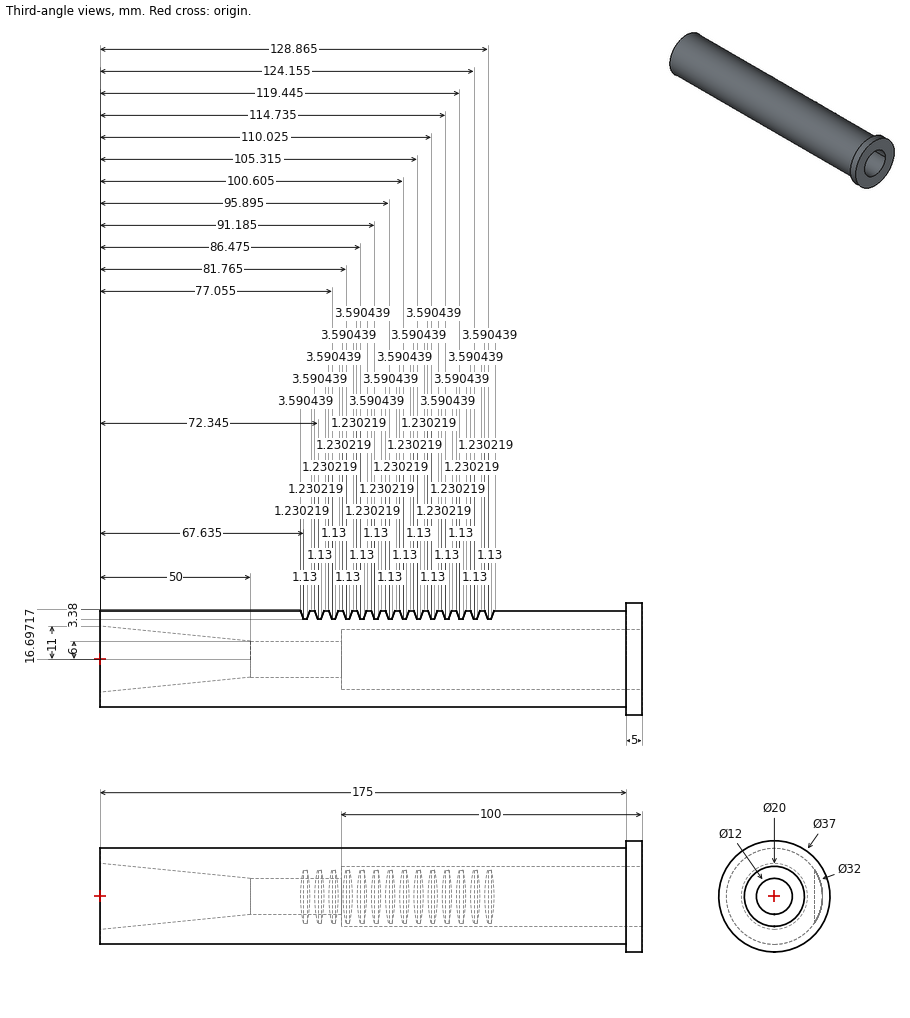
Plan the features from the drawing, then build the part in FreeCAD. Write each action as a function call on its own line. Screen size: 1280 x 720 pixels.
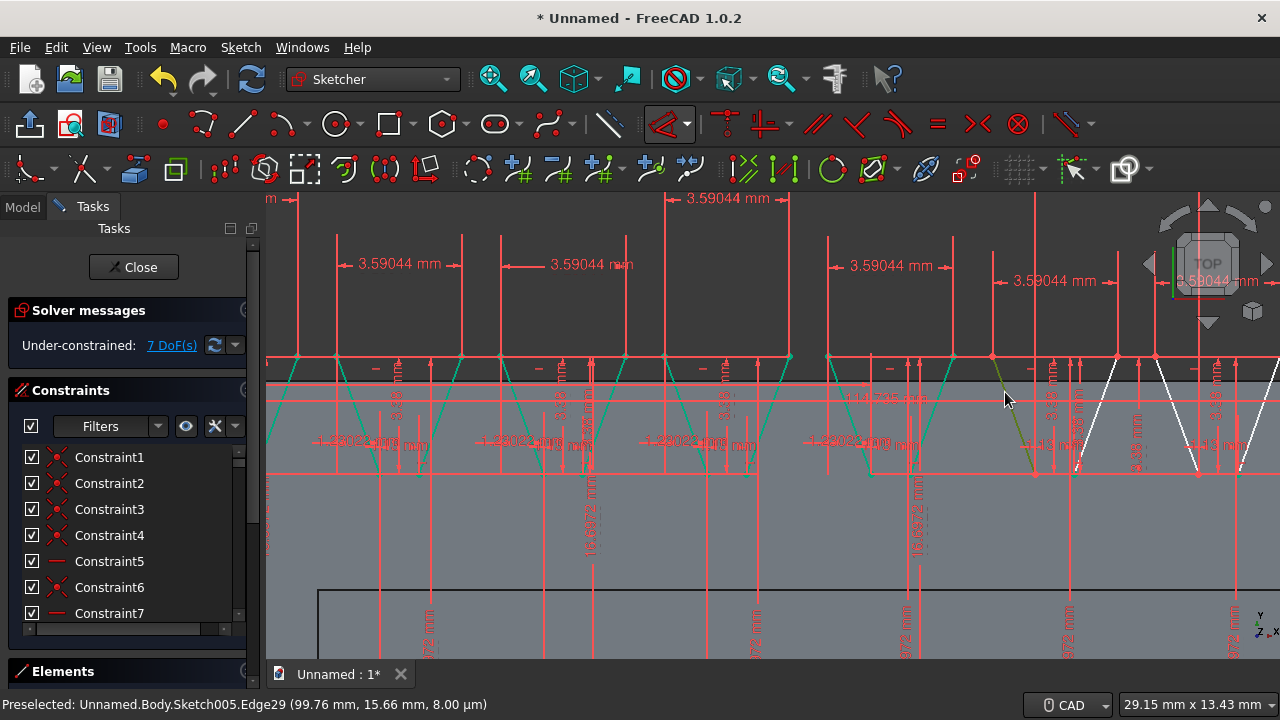
click(690, 124)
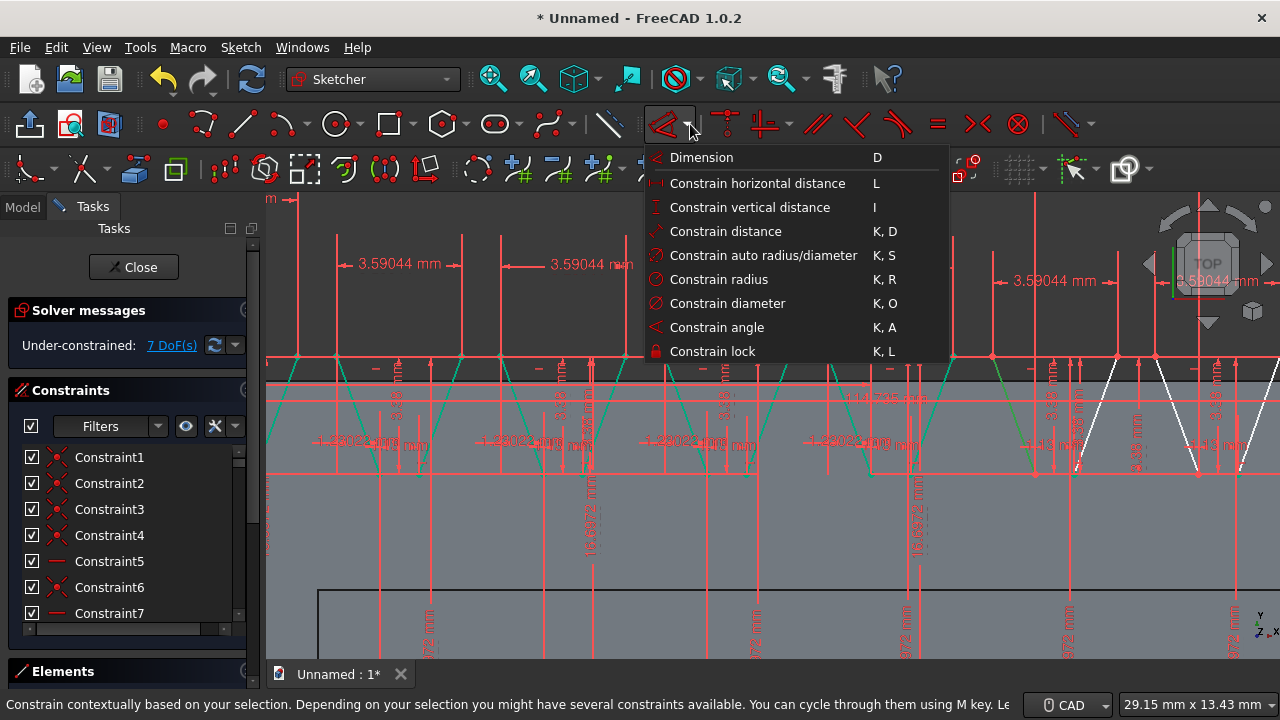
click(797, 183)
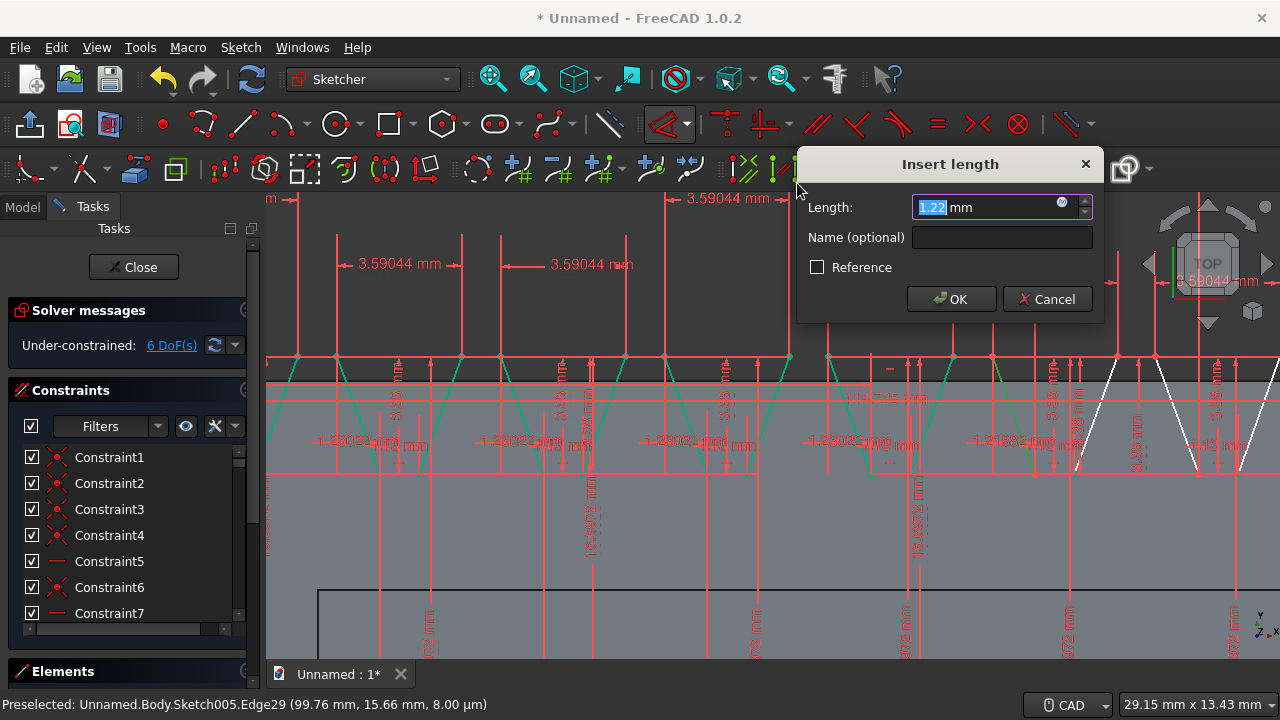
text(1.230219)
key(Return)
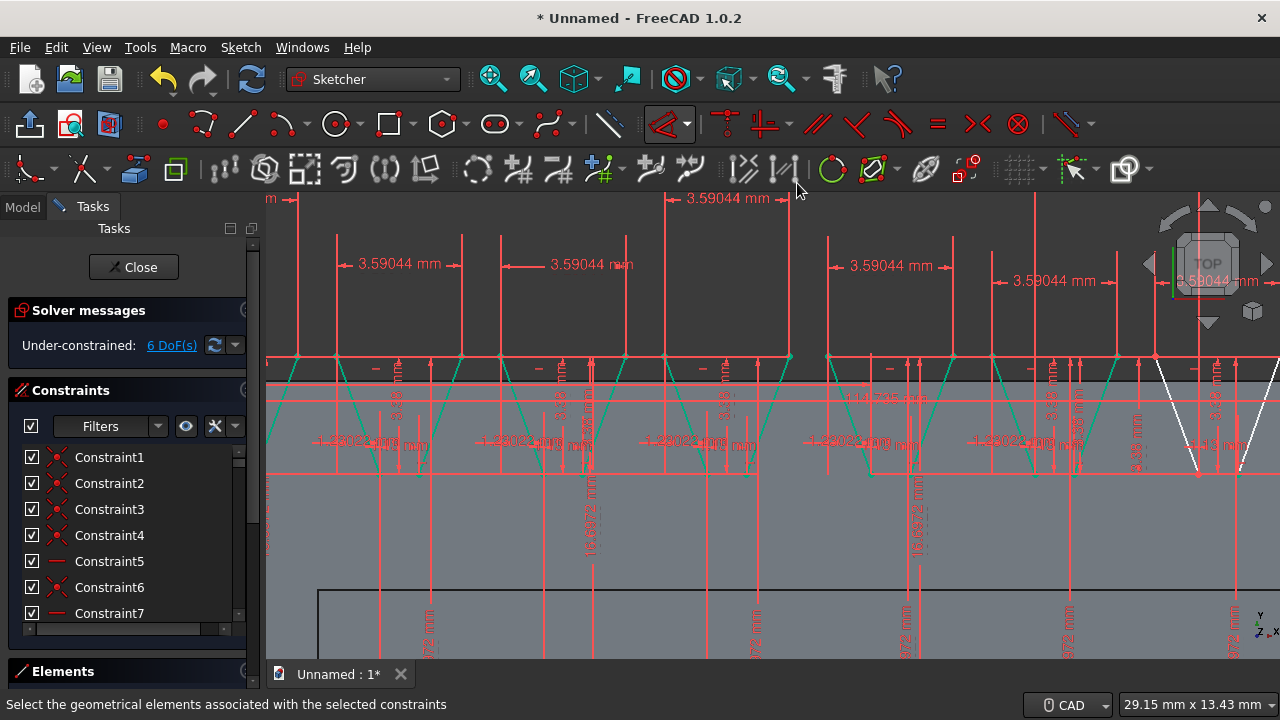
scroll(843, 391, down, 10)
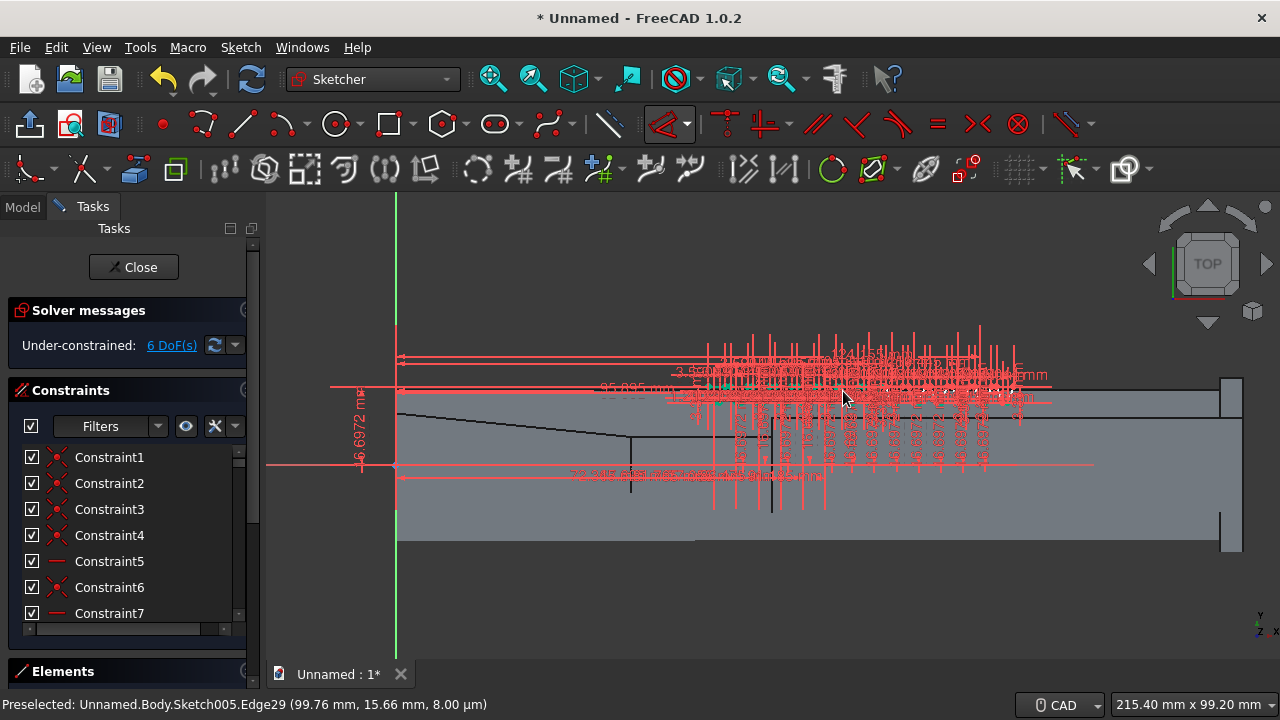
scroll(888, 391, up, 10)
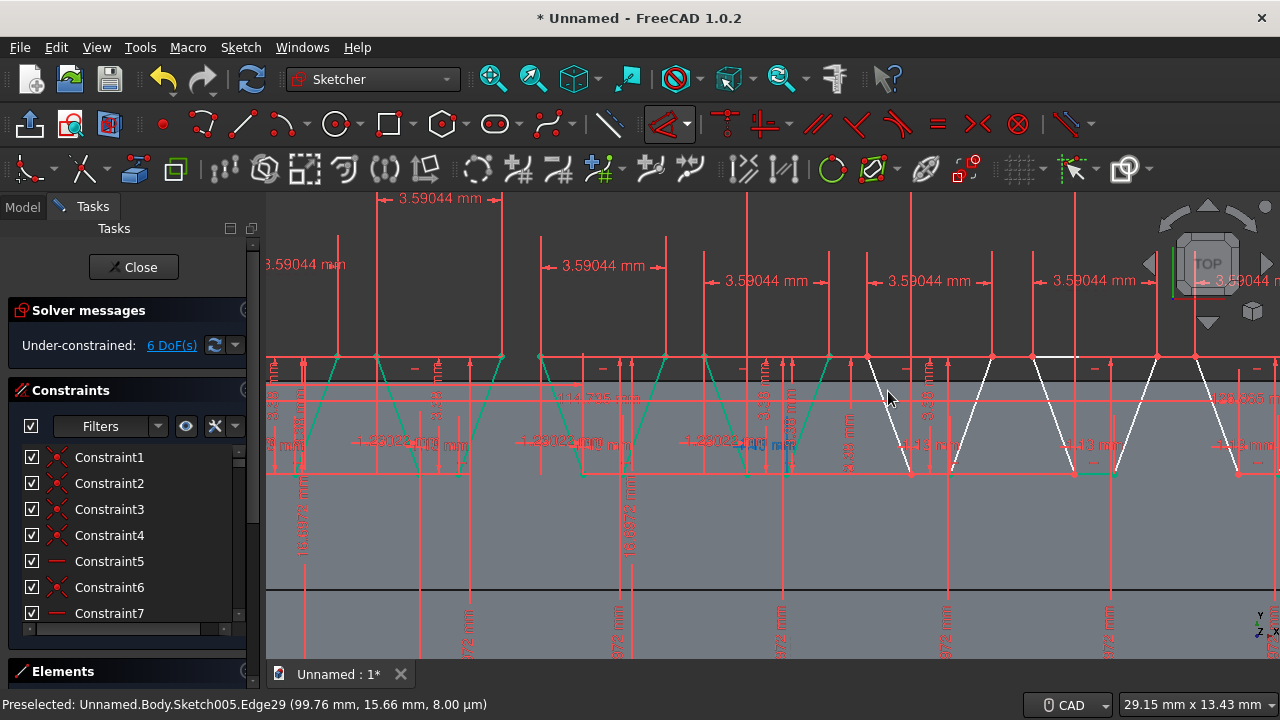
click(880, 392)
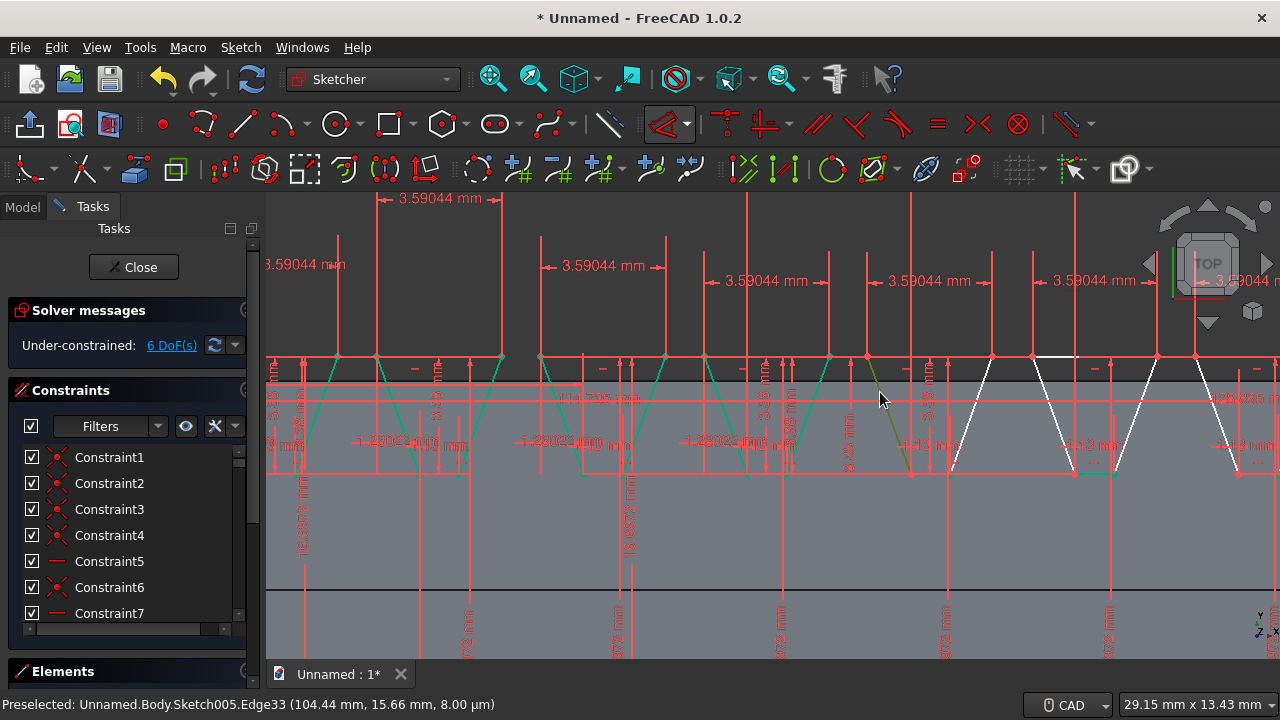
key(l)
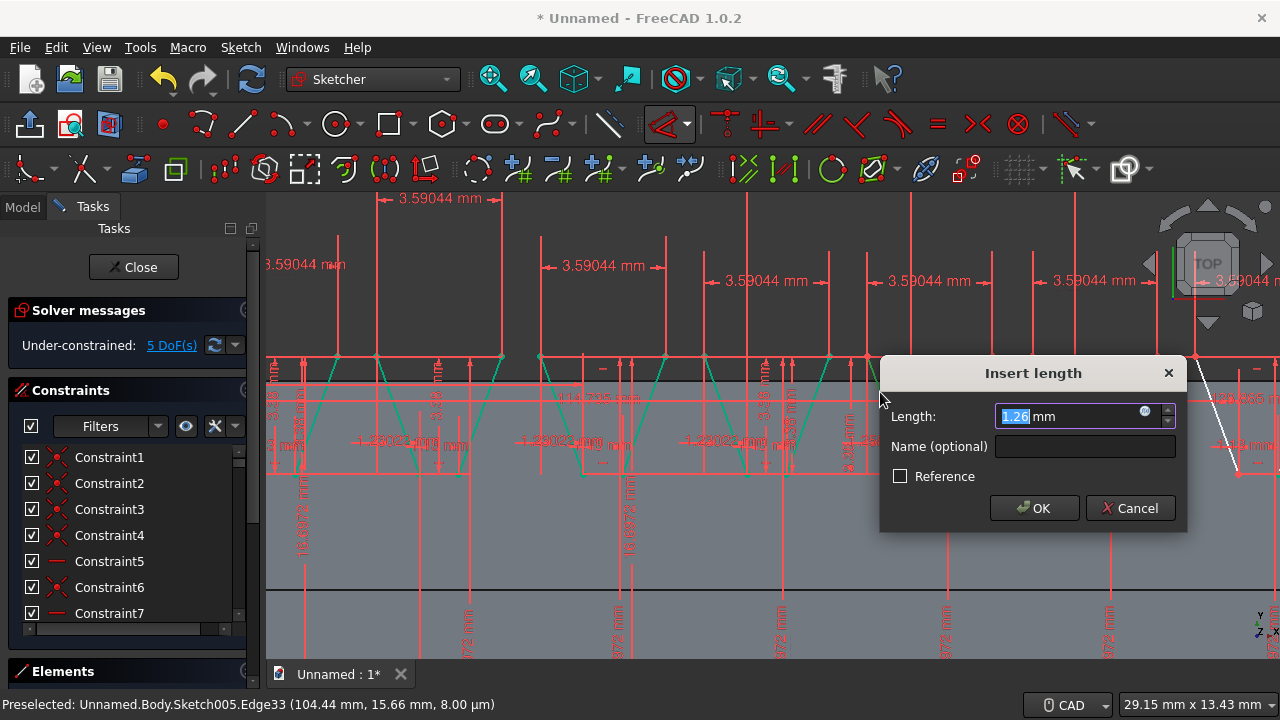
text(1.230219)
key(Return)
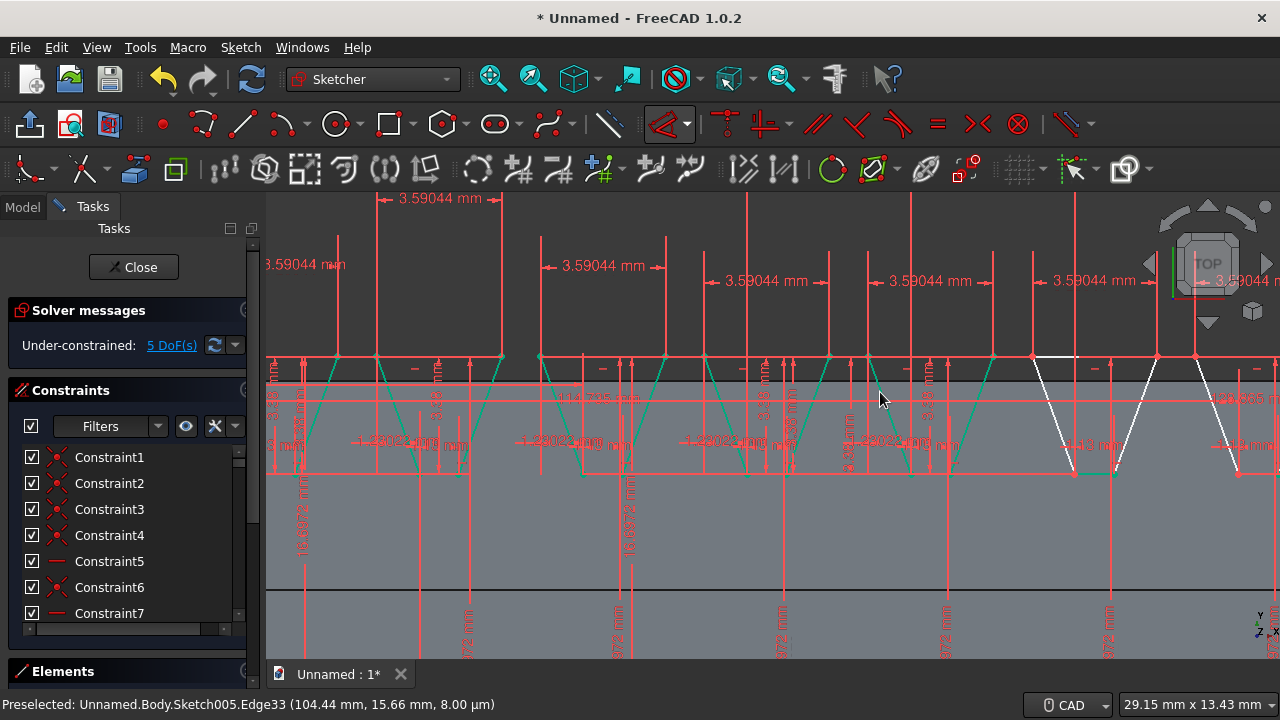
click(1045, 392)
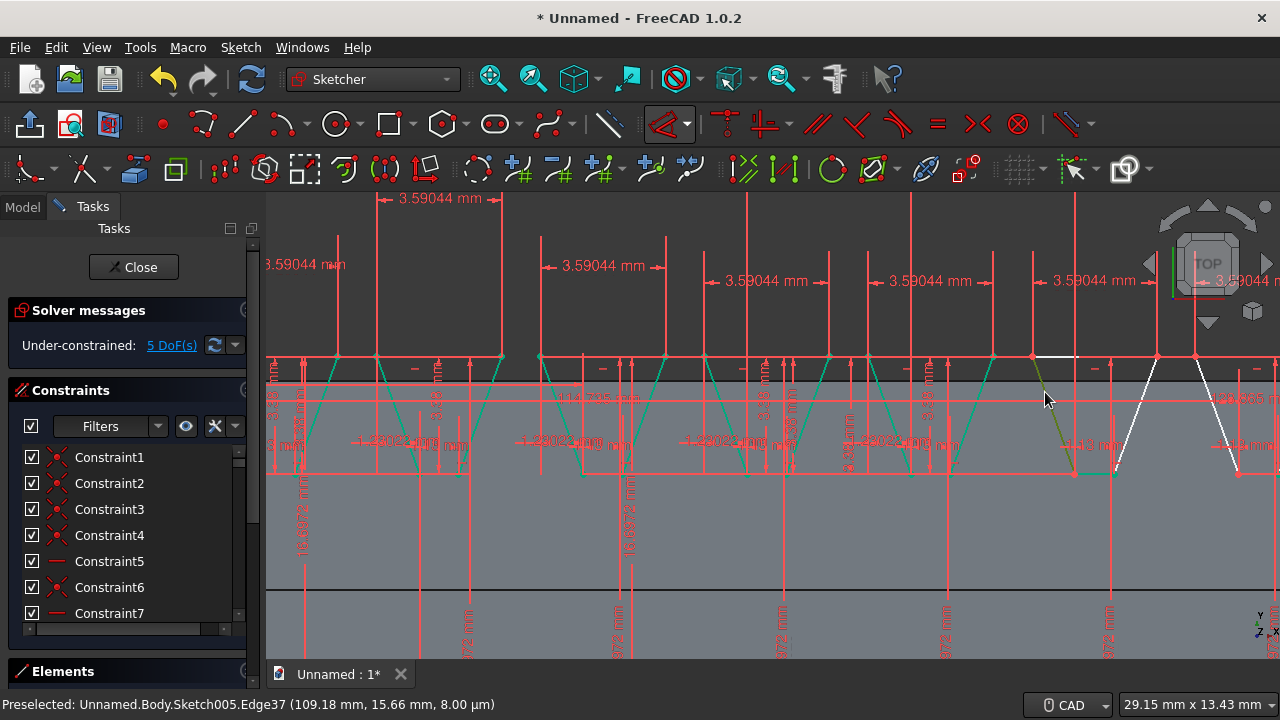
click(690, 124)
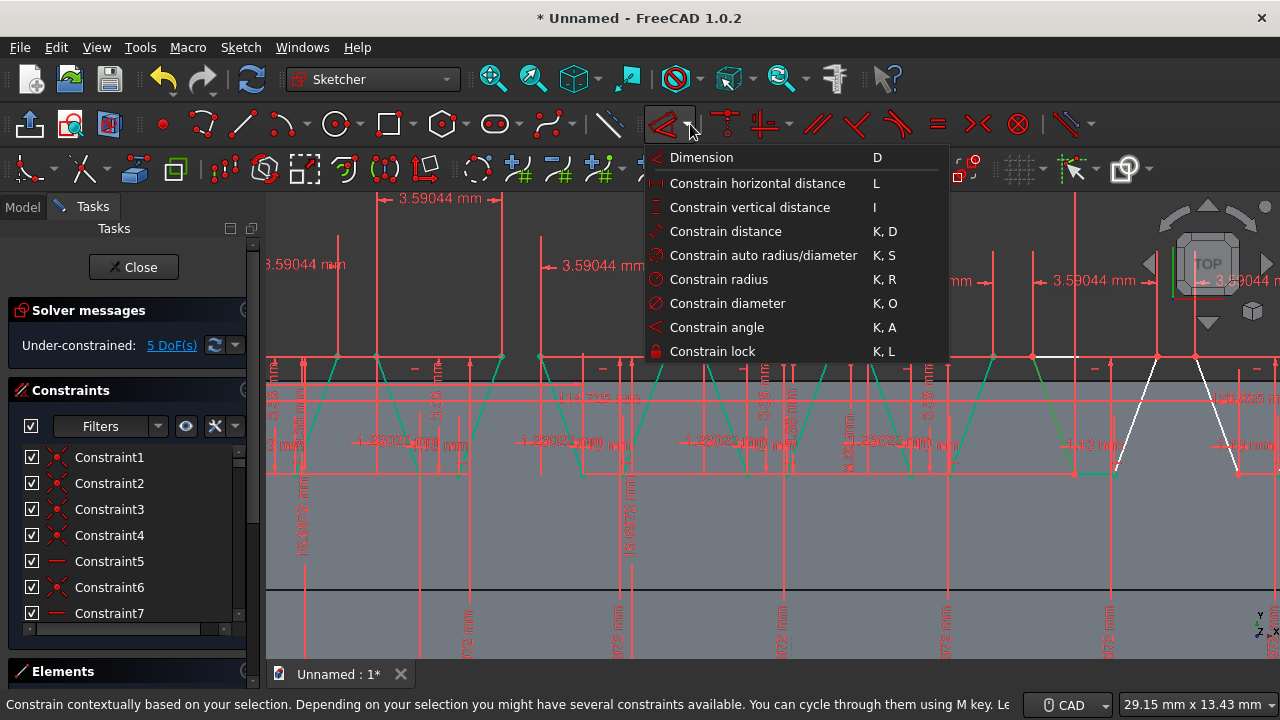
click(797, 183)